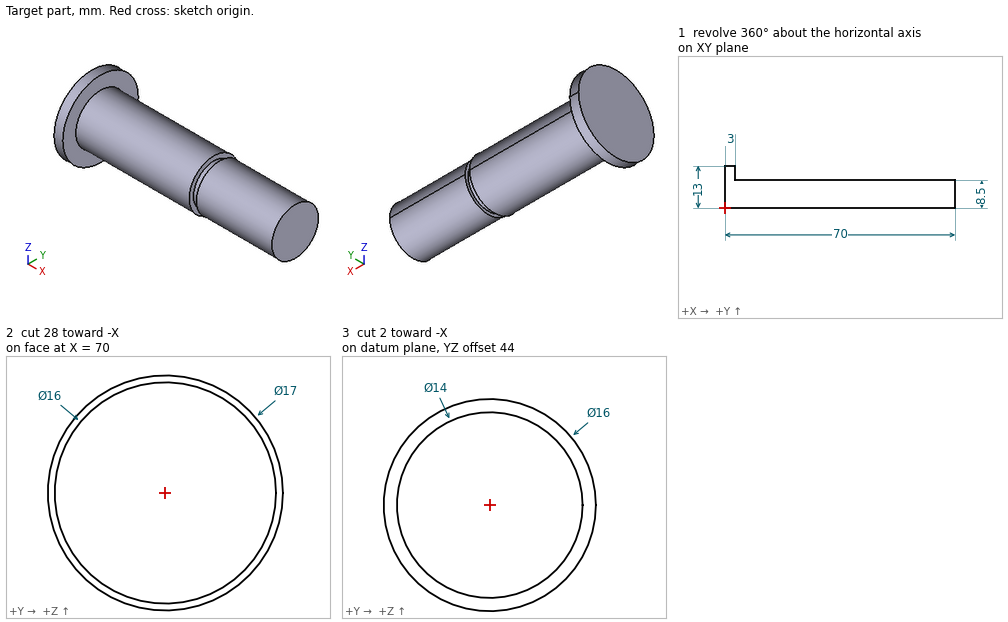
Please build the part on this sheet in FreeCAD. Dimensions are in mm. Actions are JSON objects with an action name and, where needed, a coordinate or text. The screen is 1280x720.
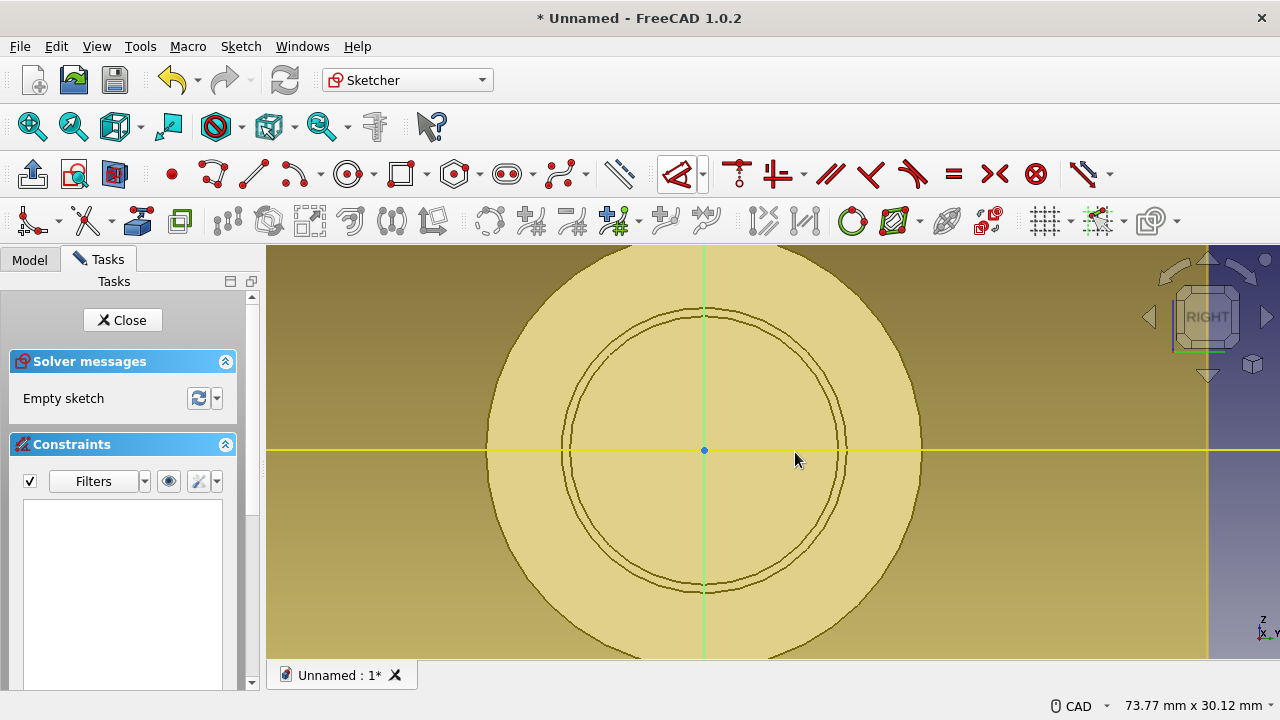
{"action": "key", "text": "g c"}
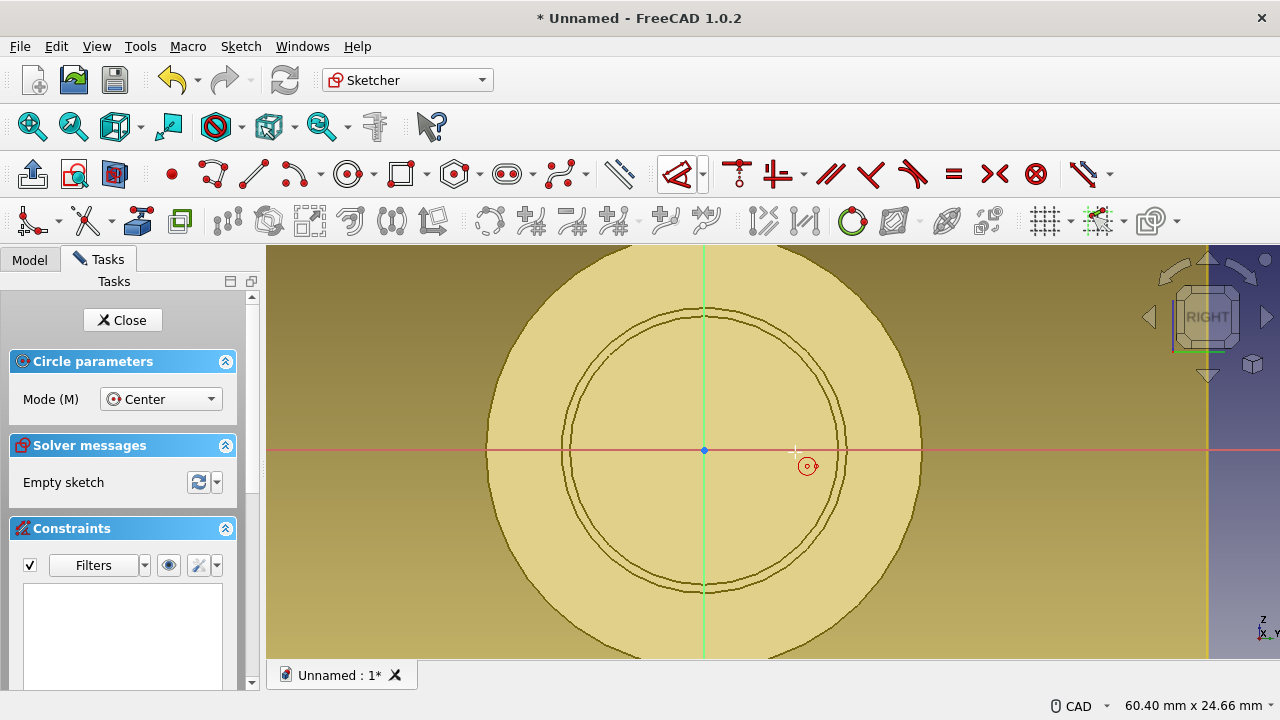
{"action": "left_click", "coordinate": [704, 450]}
{"action": "mouse_move", "coordinate": [799, 355]}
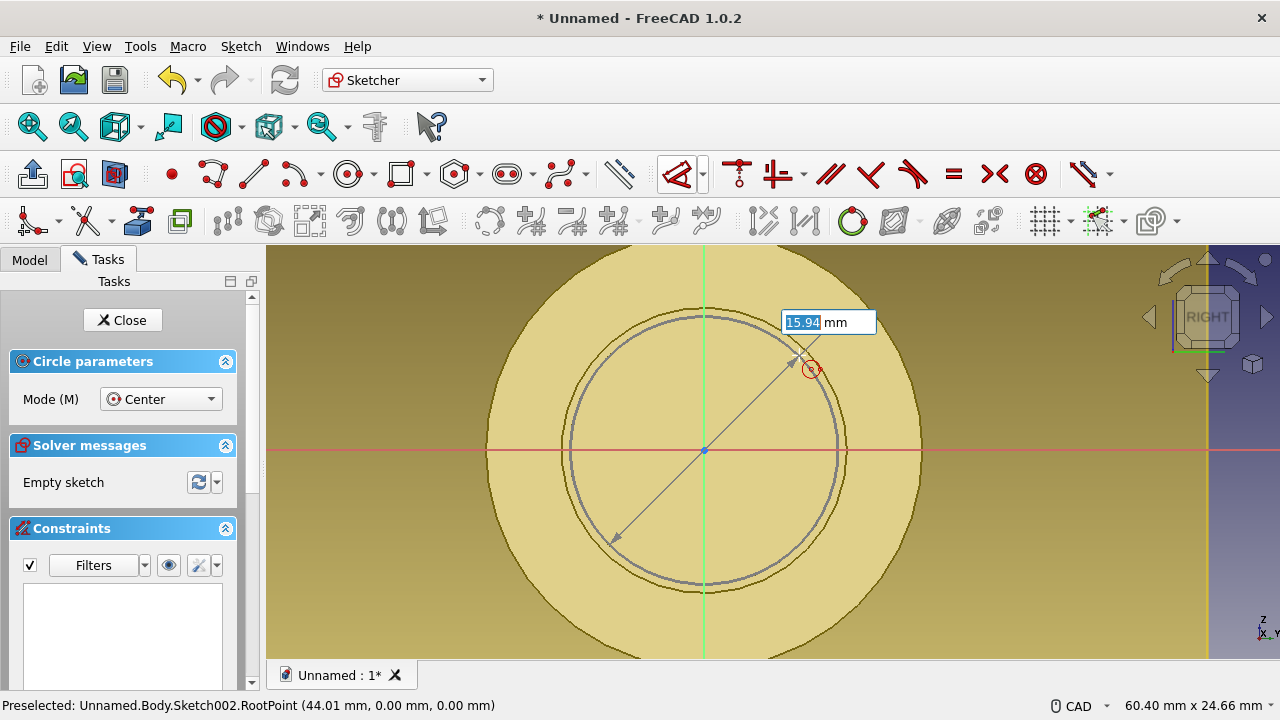
{"action": "type", "text": "16"}
{"action": "key", "text": "Return"}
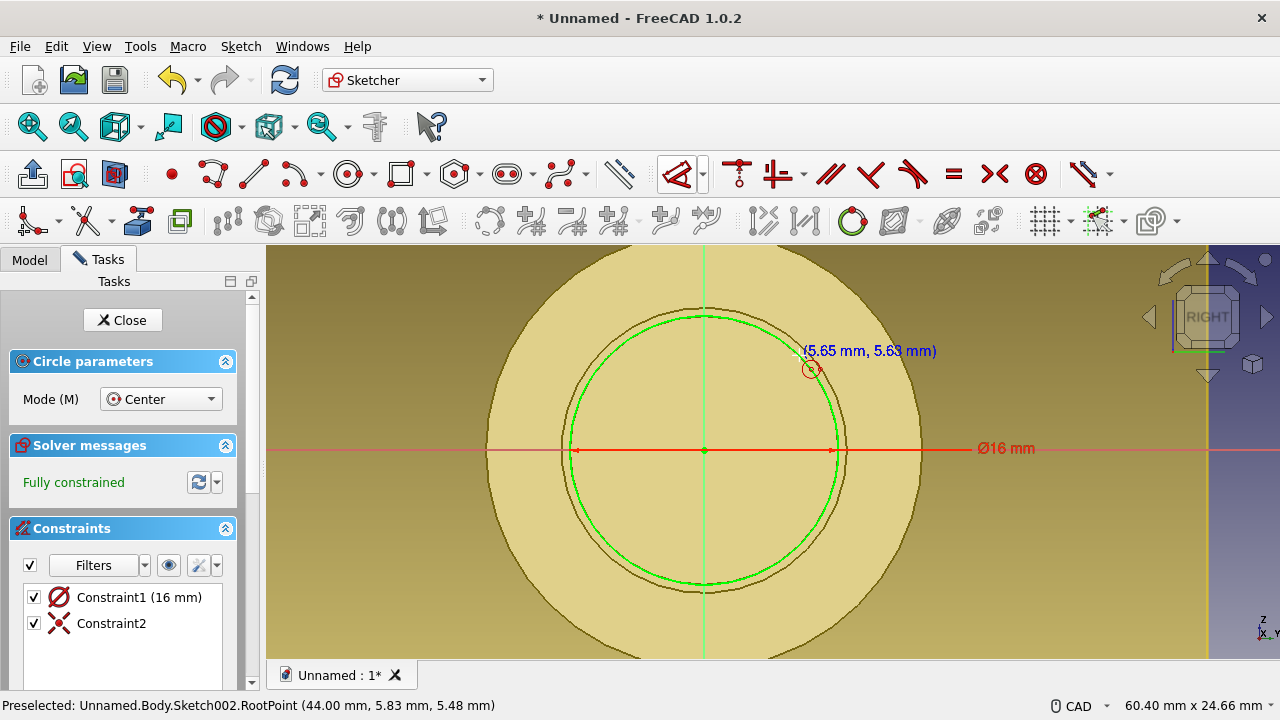
{"action": "left_click", "coordinate": [704, 450]}
{"action": "mouse_move", "coordinate": [787, 367]}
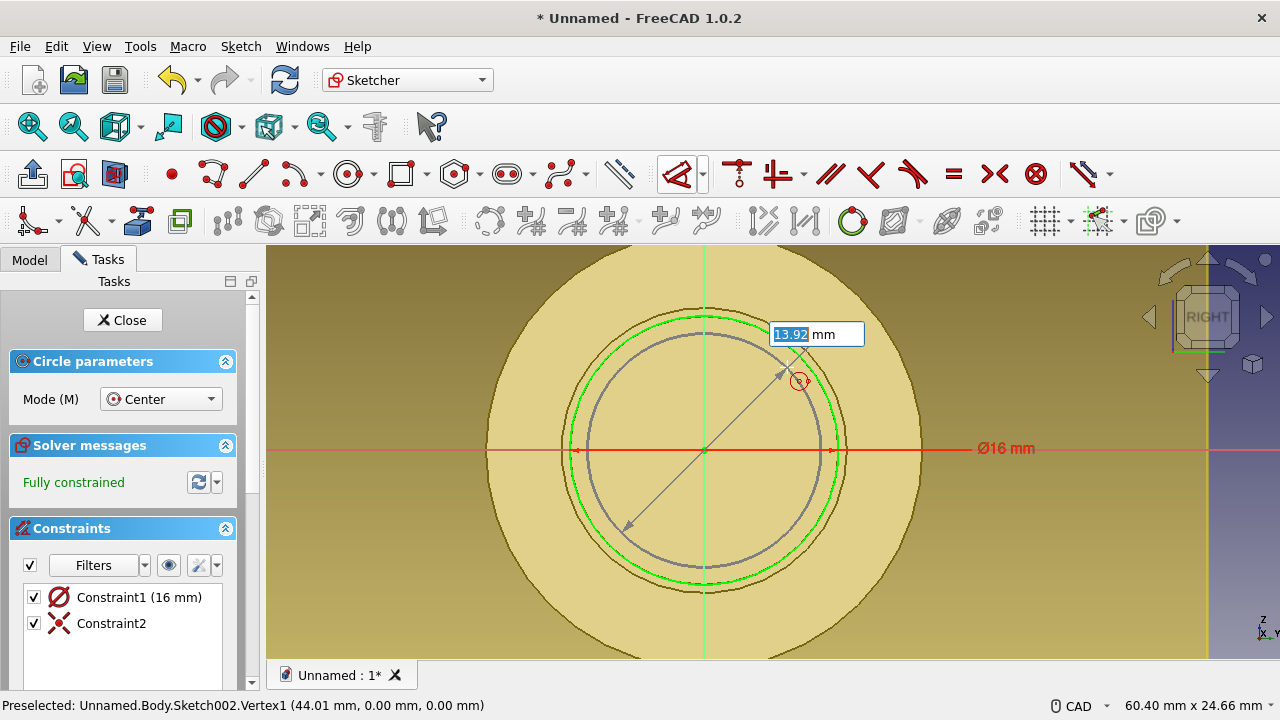
{"action": "type", "text": "14"}
{"action": "key", "text": "Return"}
{"action": "key", "text": "Escape"}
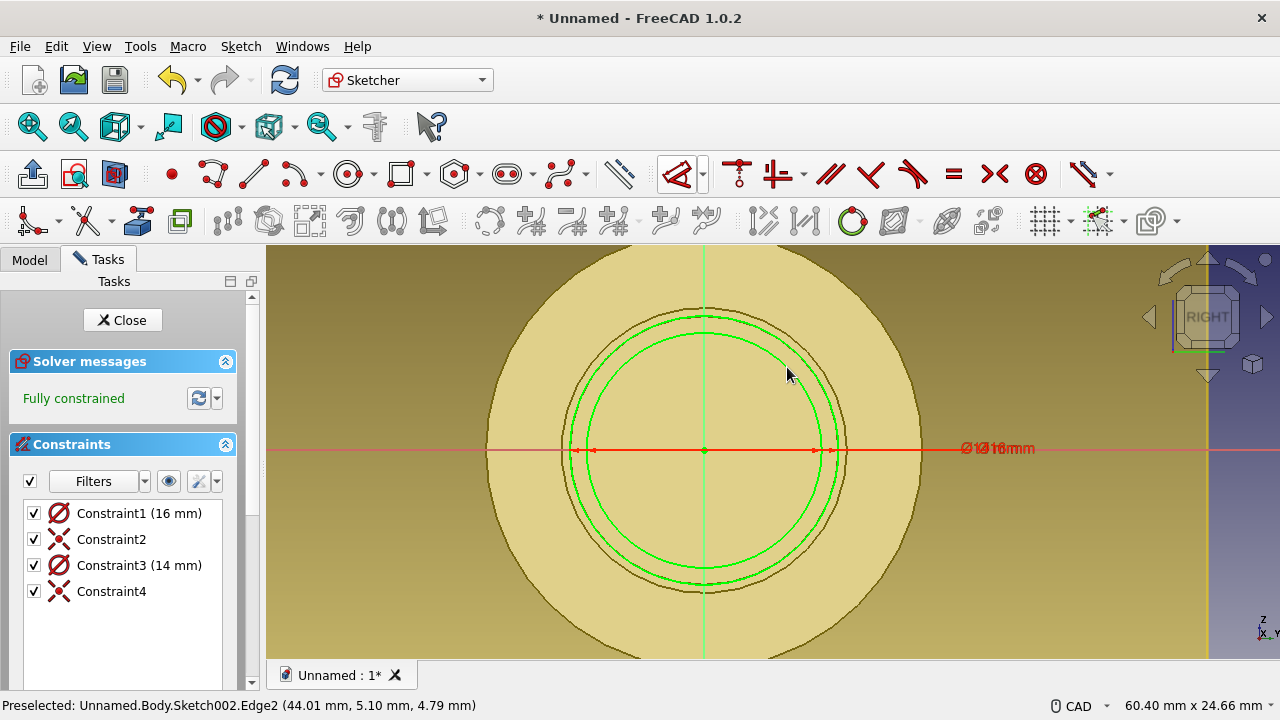
{"action": "left_click", "coordinate": [123, 320]}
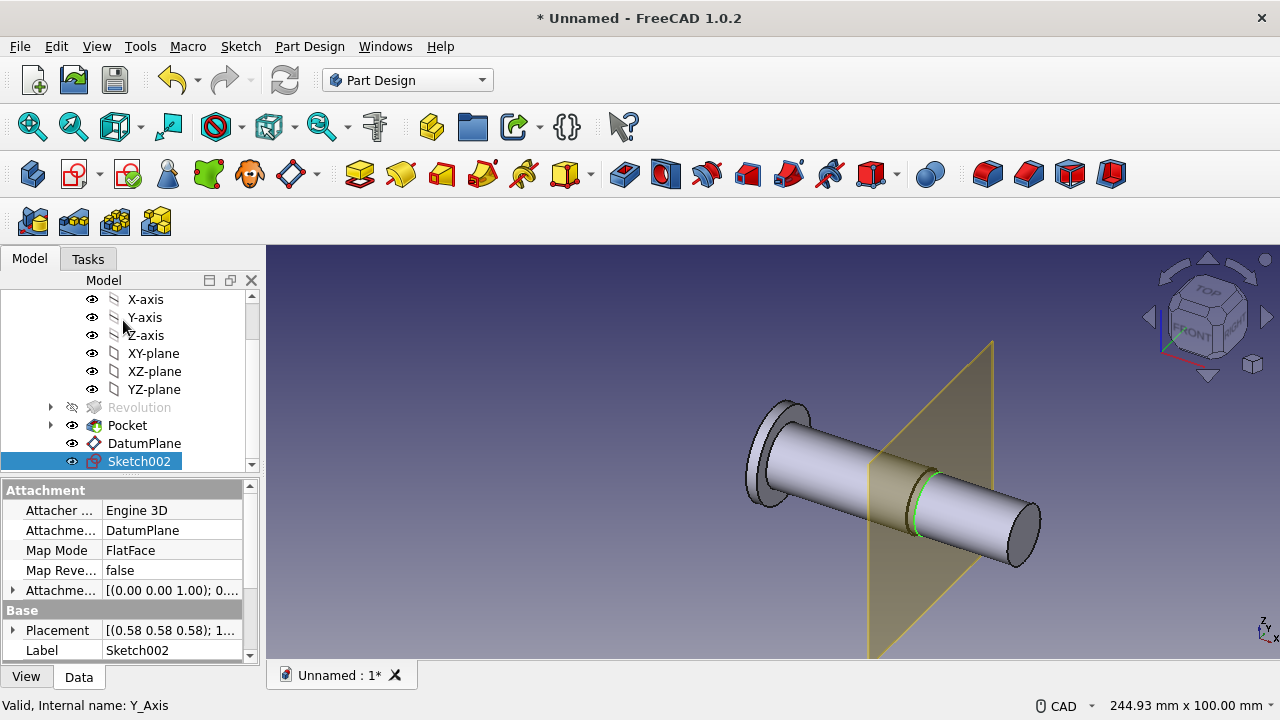
{"action": "left_click", "coordinate": [625, 174]}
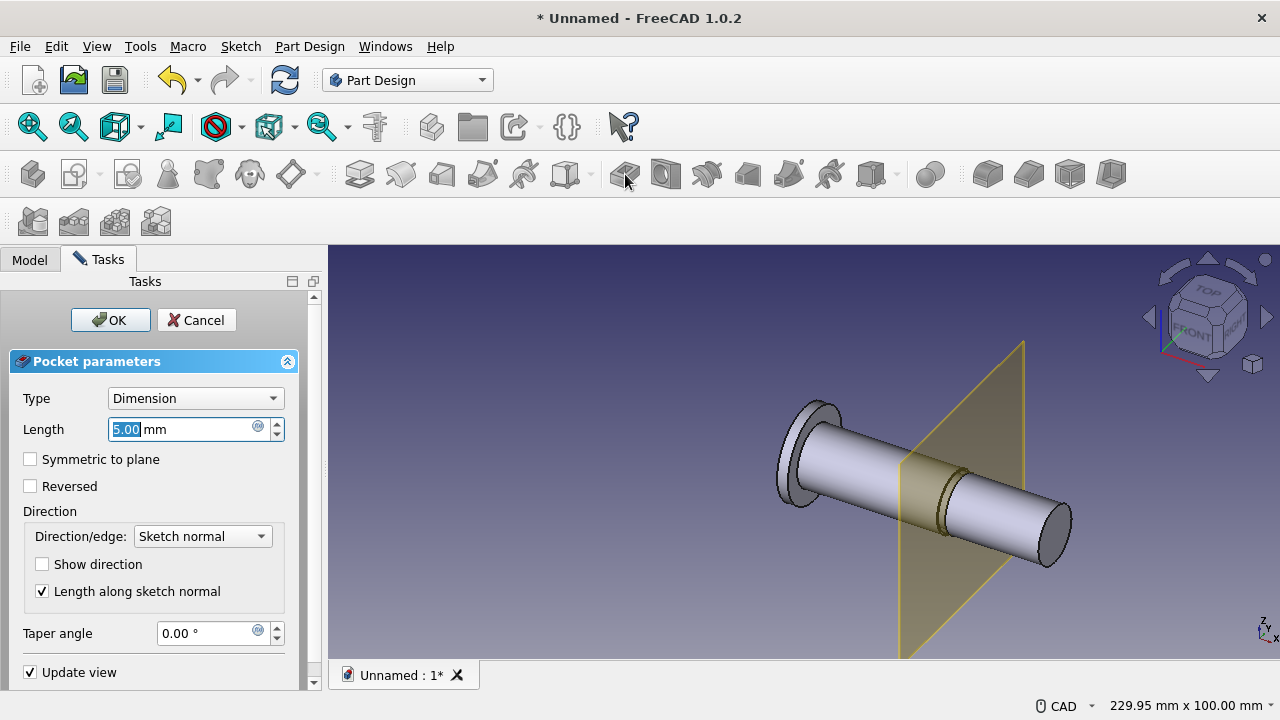
{"action": "type", "text": "2"}
{"action": "key", "text": "Tab"}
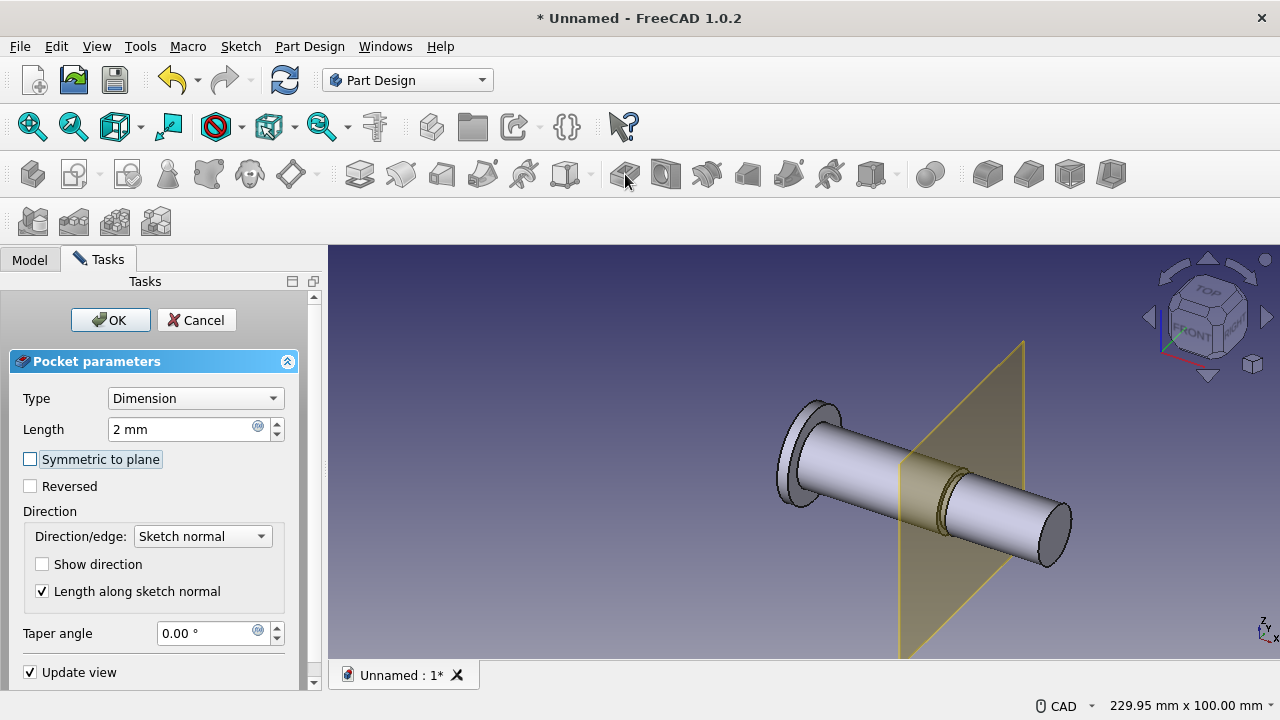
{"action": "left_click", "coordinate": [111, 320]}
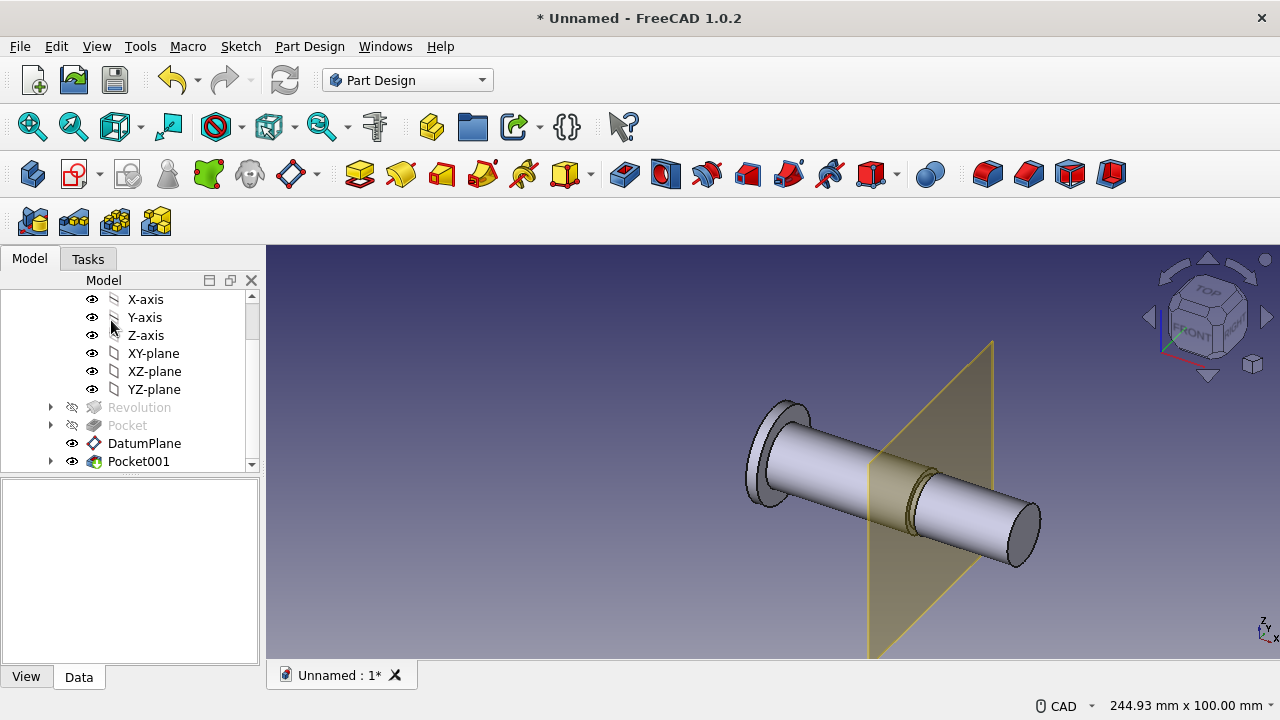
{"action": "left_click", "coordinate": [117, 443]}
{"action": "key", "text": "space"}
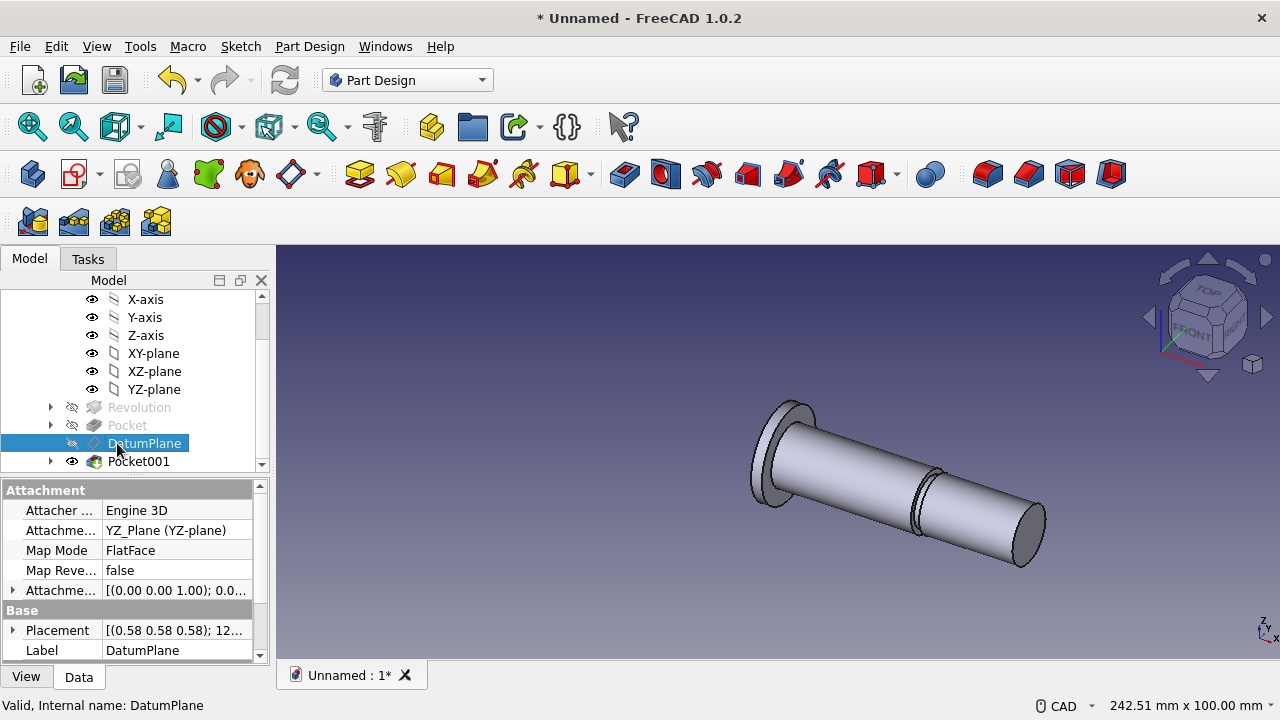
{"action": "key", "text": "0"}